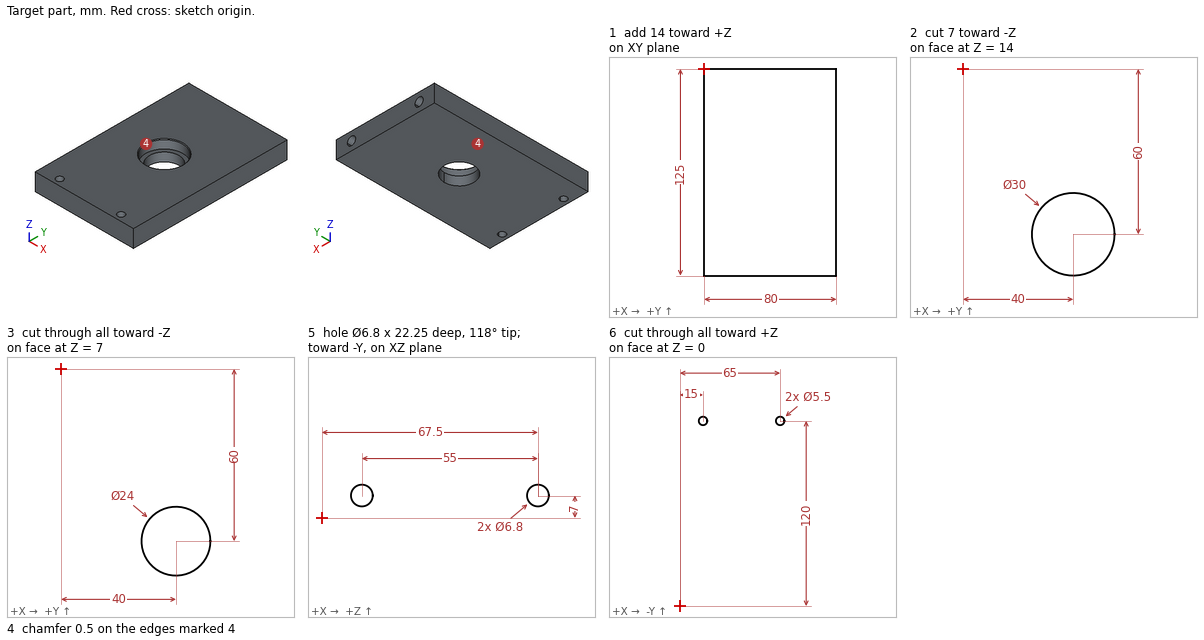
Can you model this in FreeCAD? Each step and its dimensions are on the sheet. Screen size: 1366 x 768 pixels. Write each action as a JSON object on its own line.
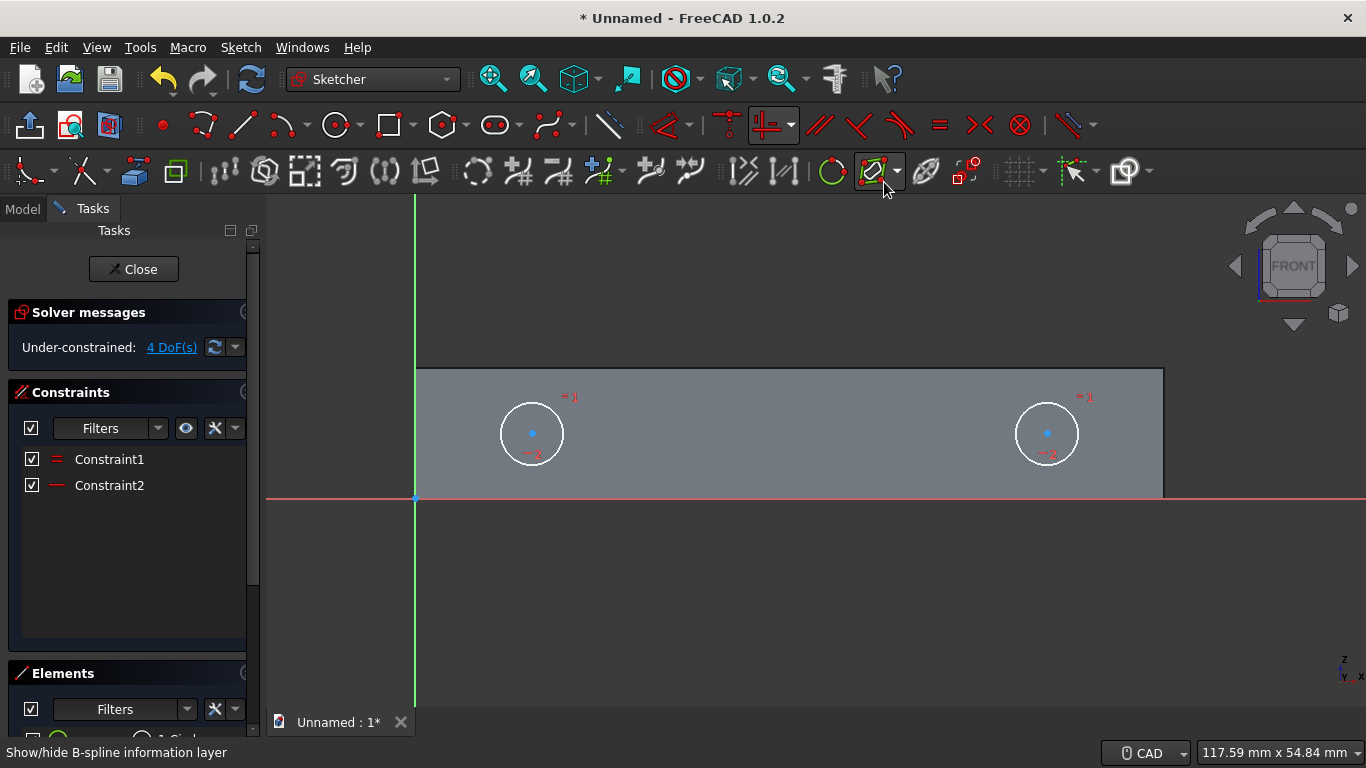
{"action": "key", "text": "d"}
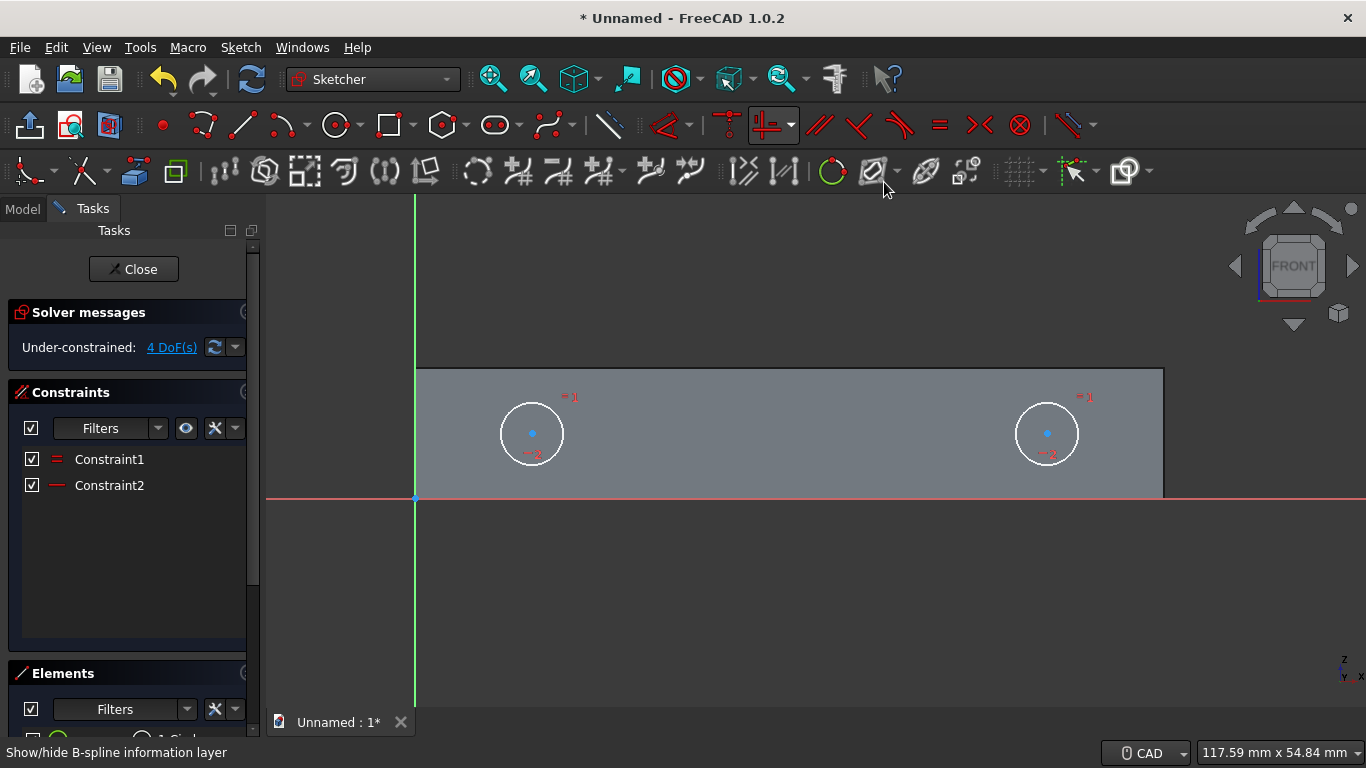
{"action": "left_click", "coordinate": [1069, 412]}
{"action": "left_click", "coordinate": [1092, 389]}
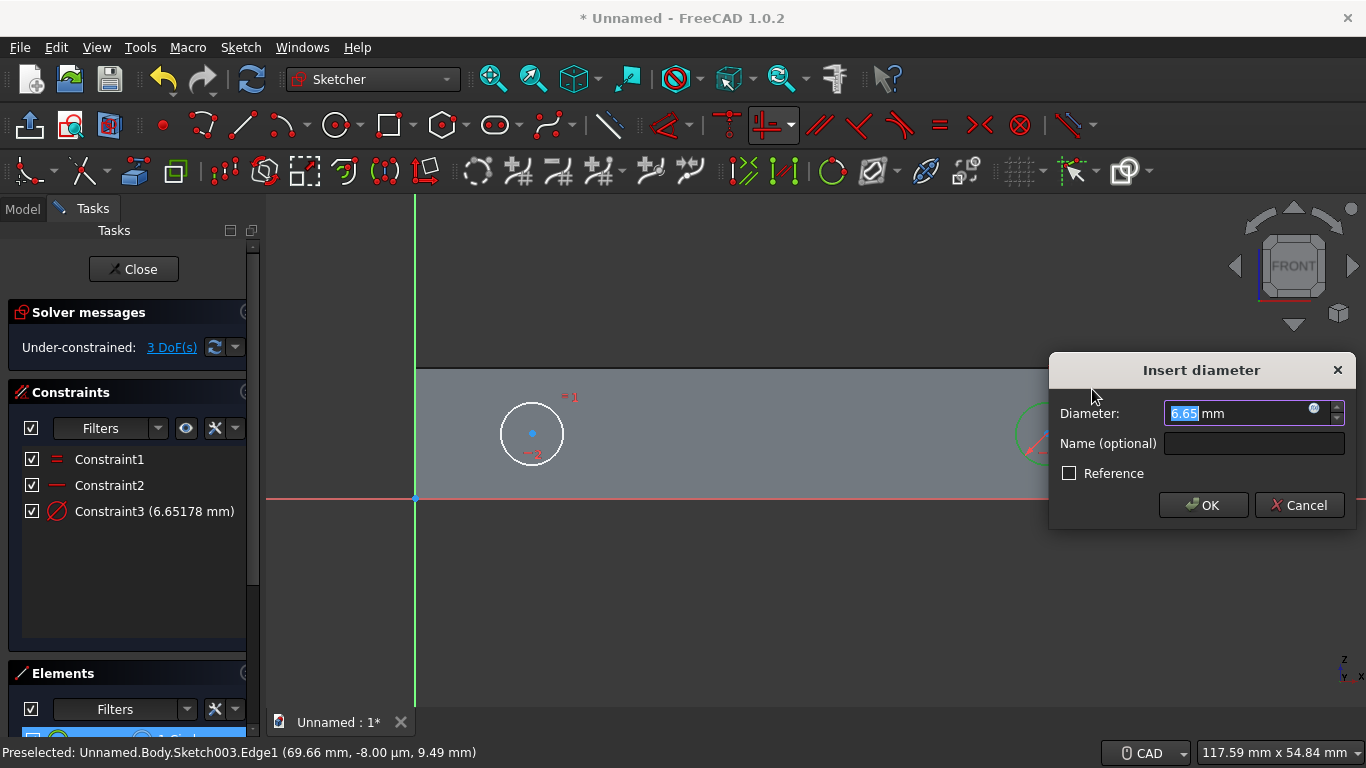
{"action": "type", "text": "6.8"}
{"action": "key", "text": "Return"}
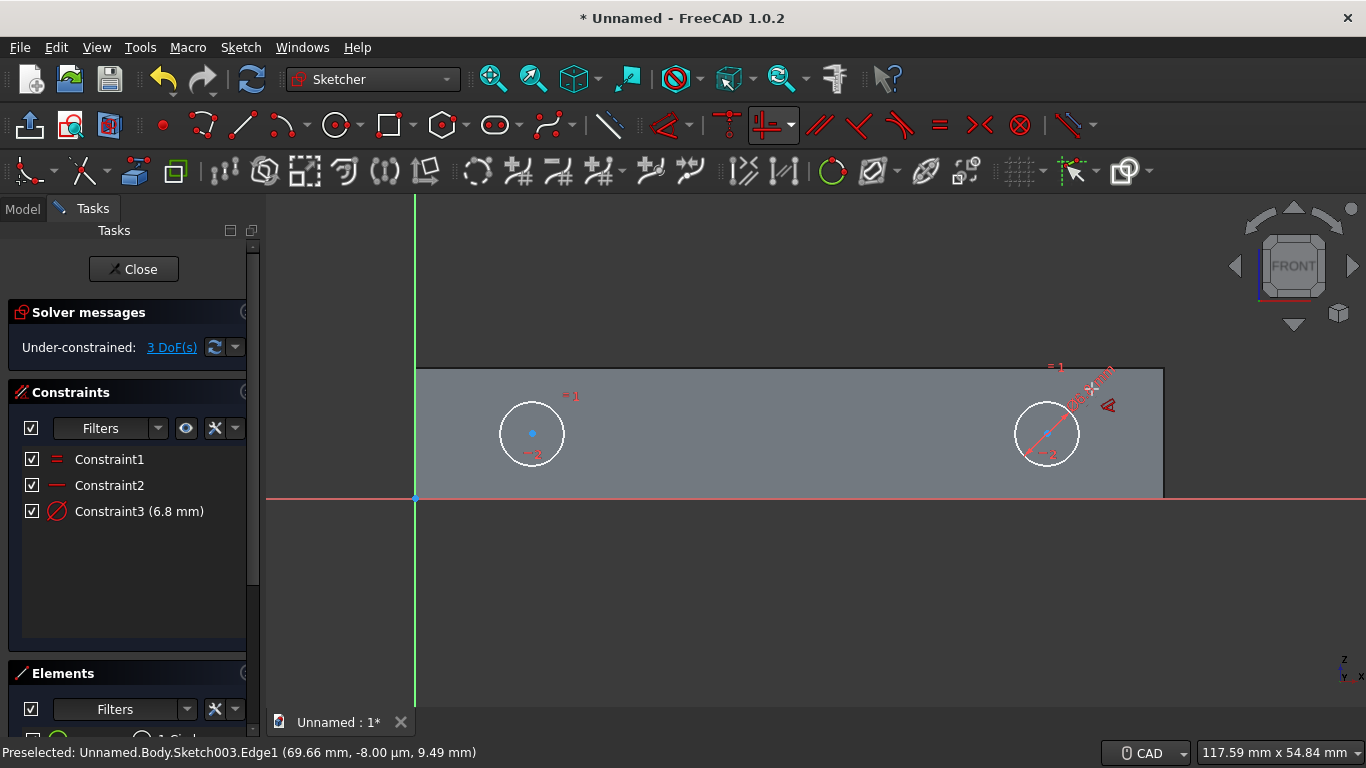
{"action": "left_click", "coordinate": [1047, 434]}
{"action": "left_click", "coordinate": [381, 466]}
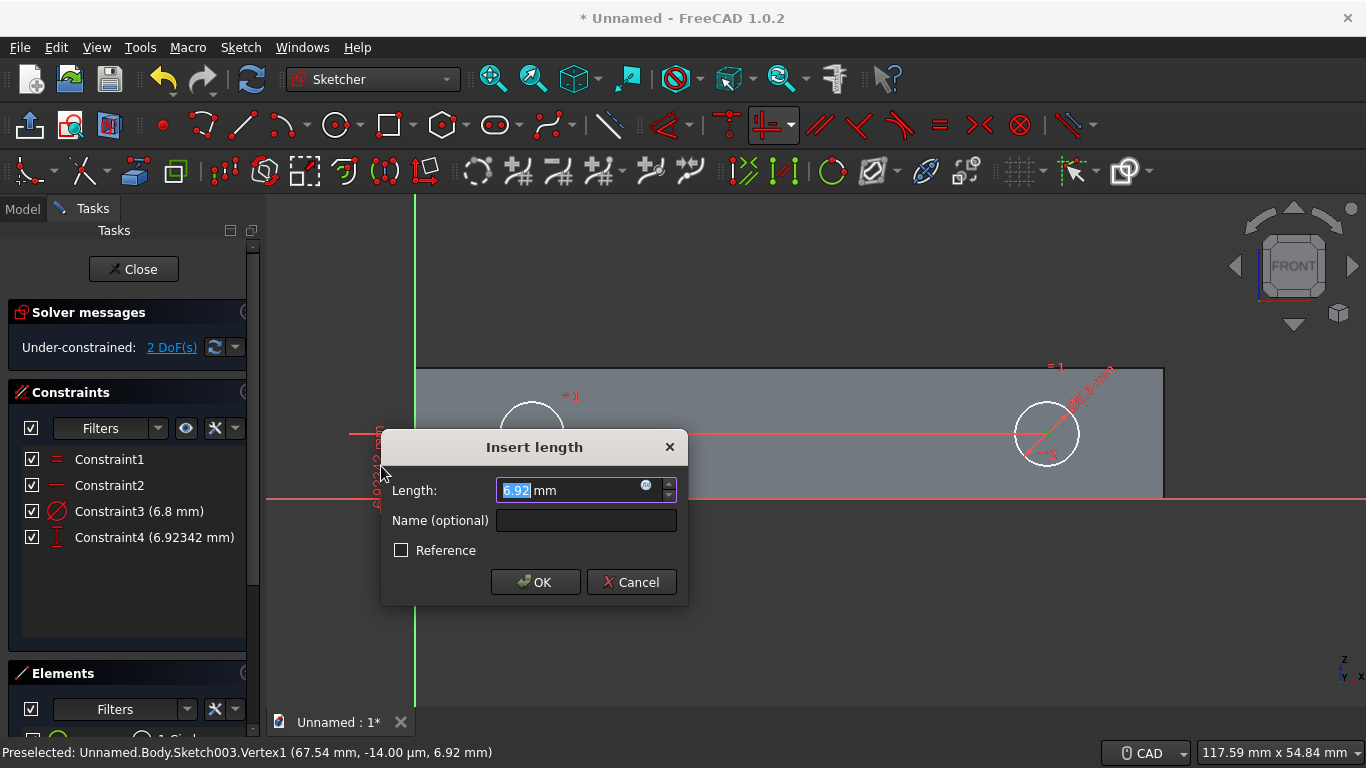
{"action": "type", "text": "7"}
{"action": "key", "text": "Return"}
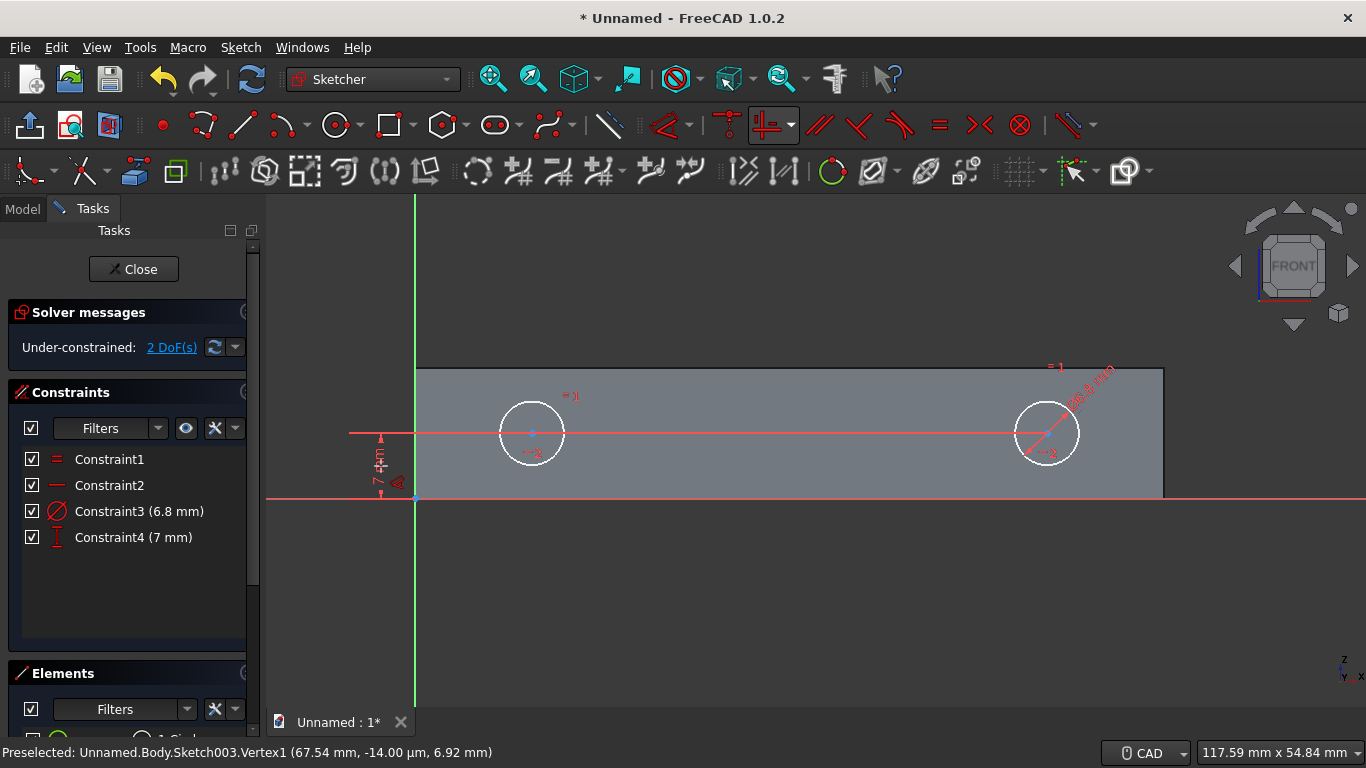
{"action": "left_click", "coordinate": [1047, 433]}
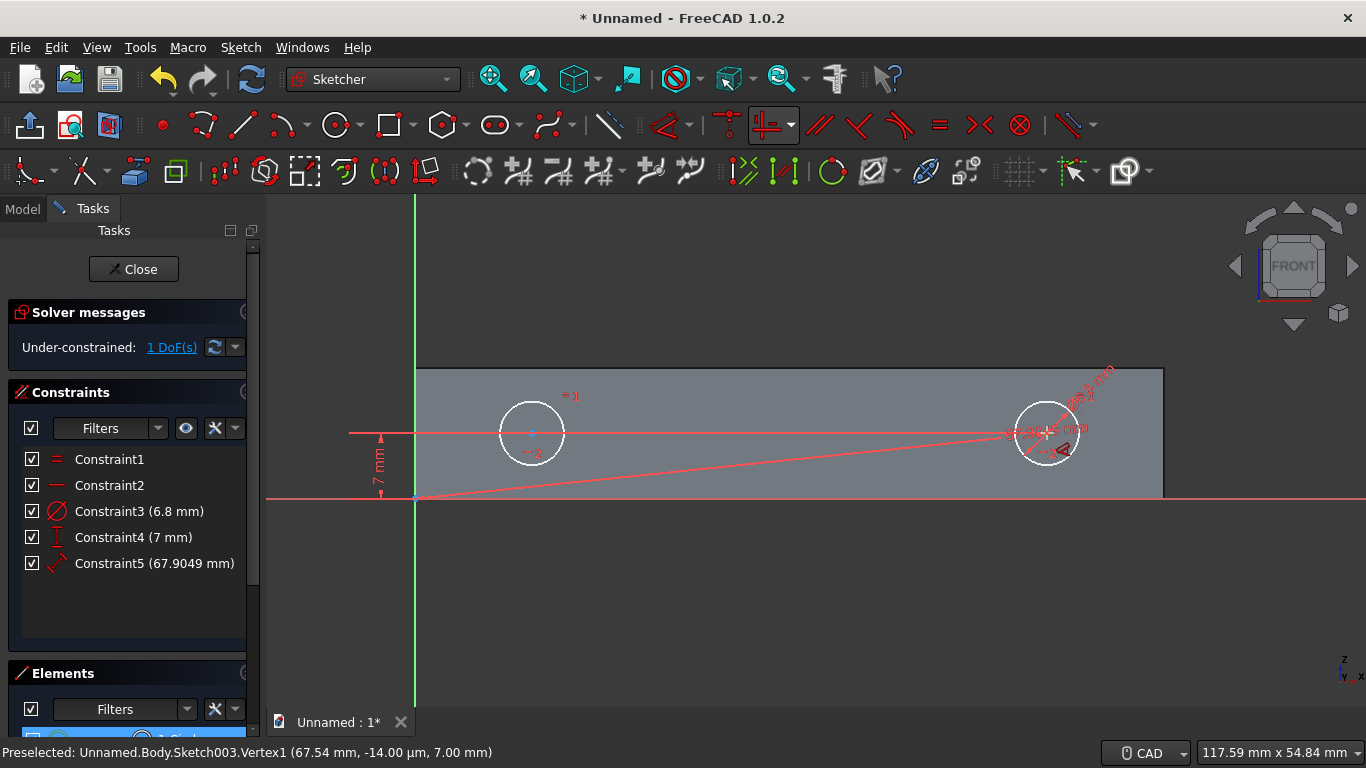
{"action": "left_click", "coordinate": [532, 433]}
{"action": "left_click", "coordinate": [789, 399]}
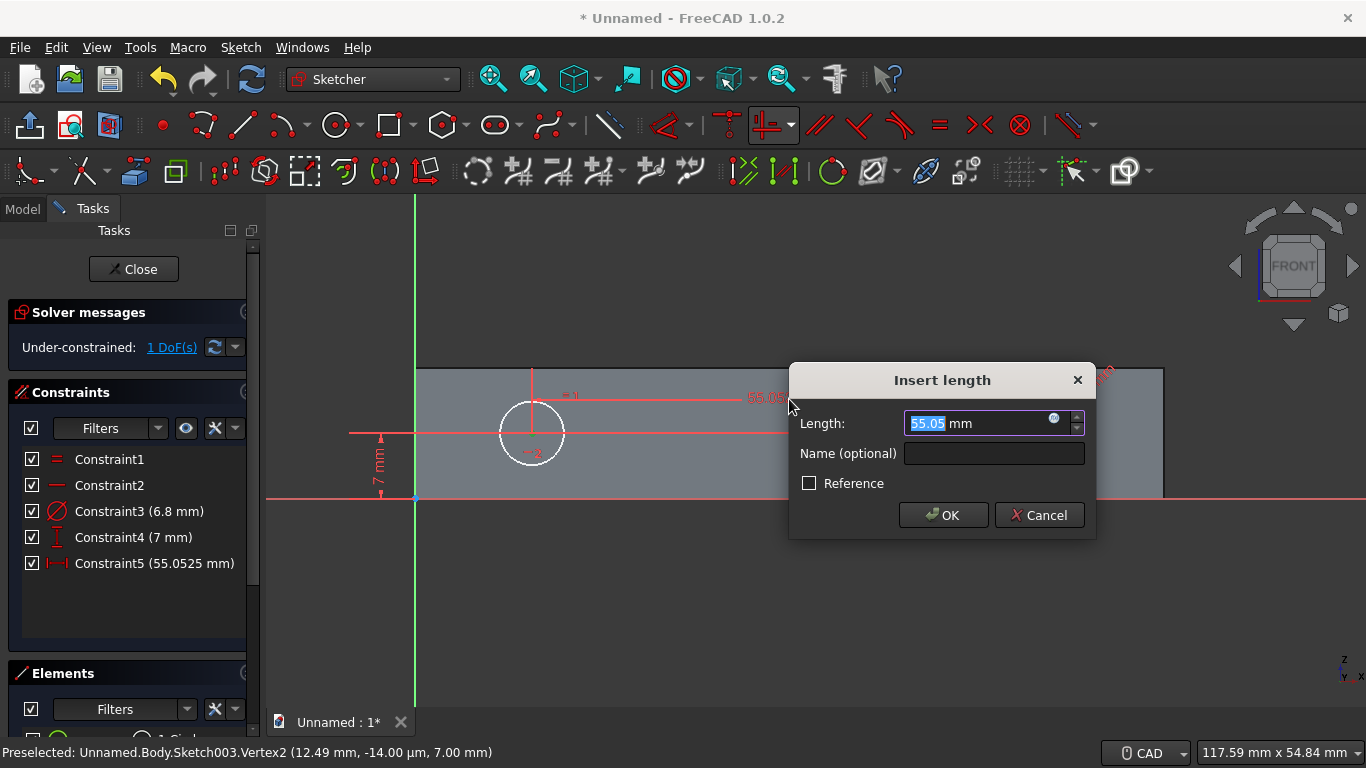
{"action": "type", "text": "55"}
{"action": "key", "text": "Return"}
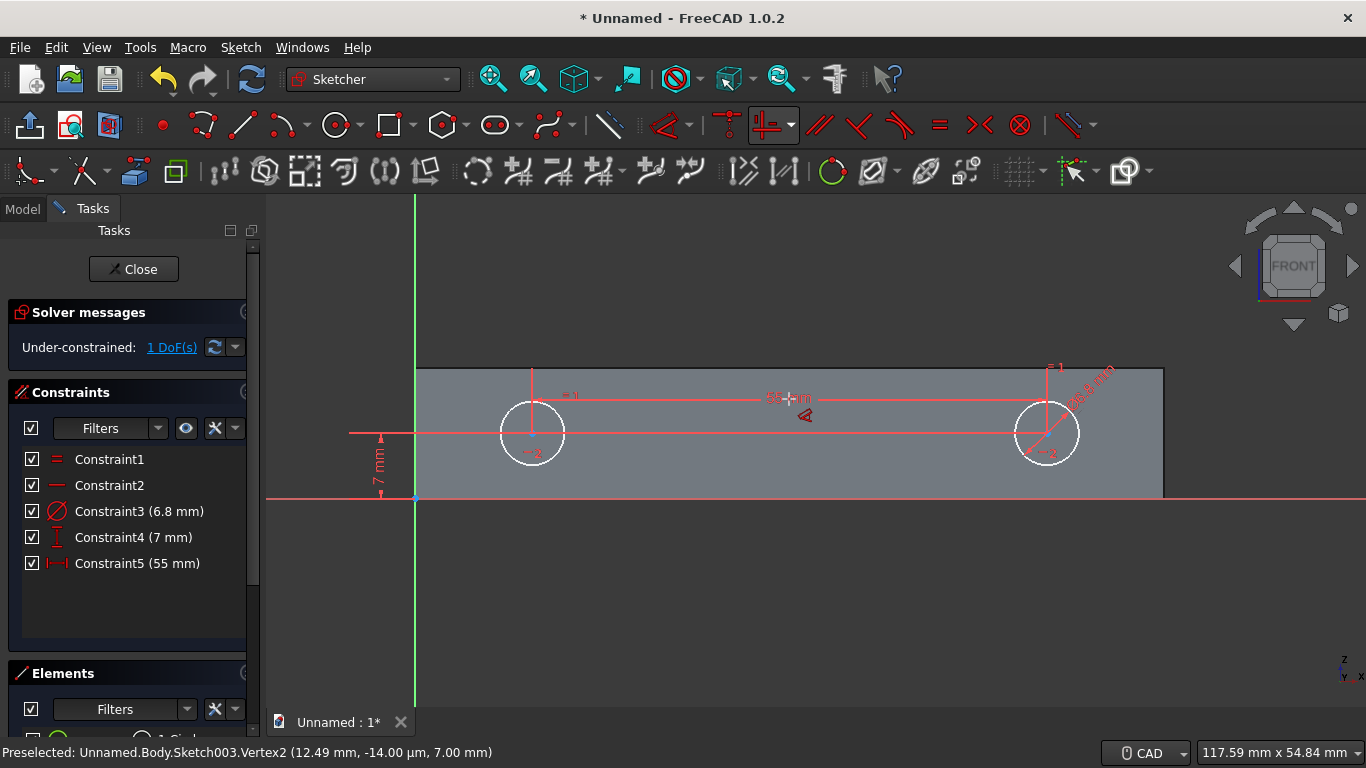
{"action": "left_click", "coordinate": [1047, 433]}
{"action": "left_click", "coordinate": [731, 533]}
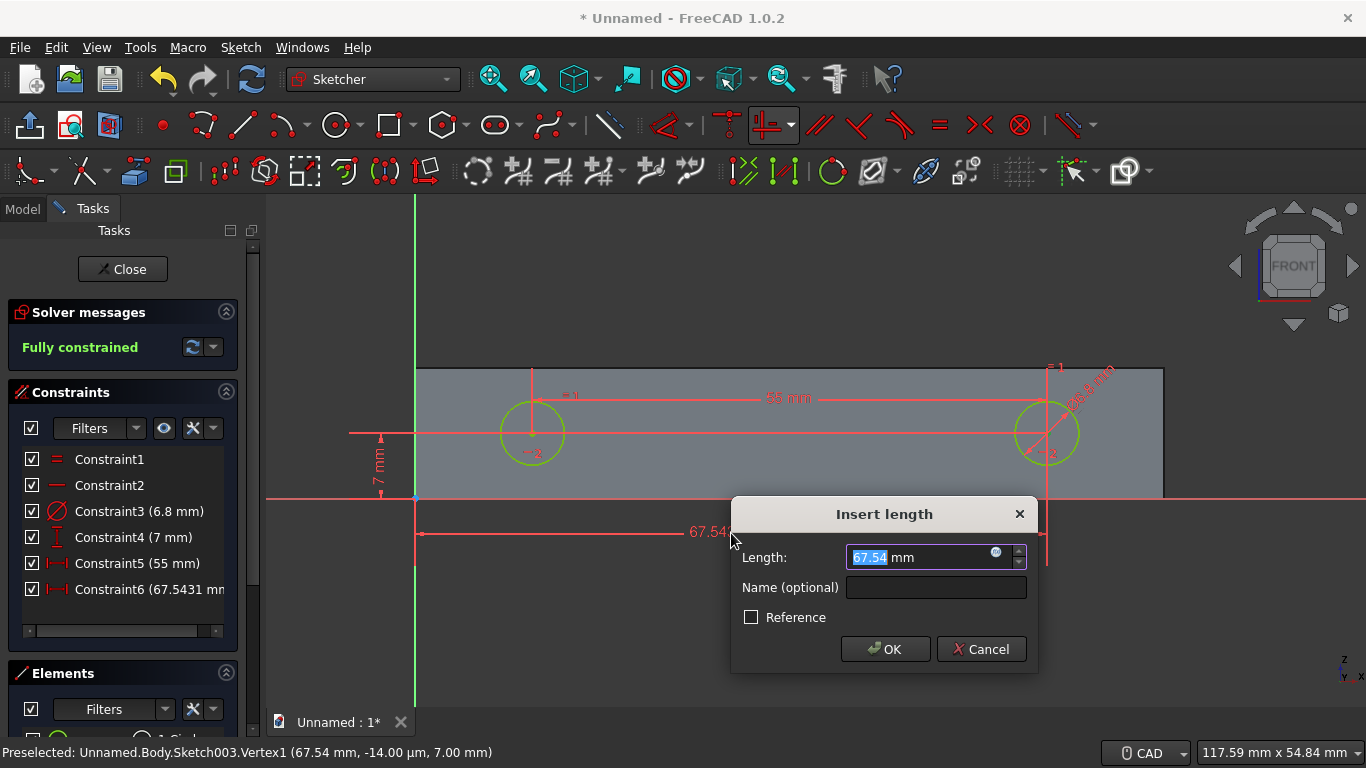
{"action": "type", "text": "67.5"}
{"action": "key", "text": "Return"}
{"action": "key", "text": "Escape"}